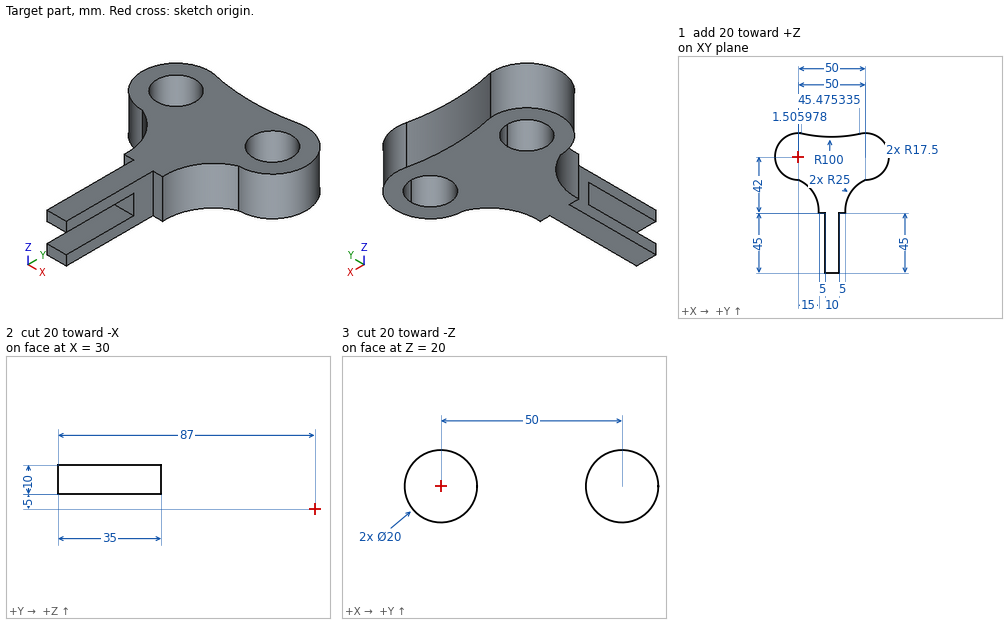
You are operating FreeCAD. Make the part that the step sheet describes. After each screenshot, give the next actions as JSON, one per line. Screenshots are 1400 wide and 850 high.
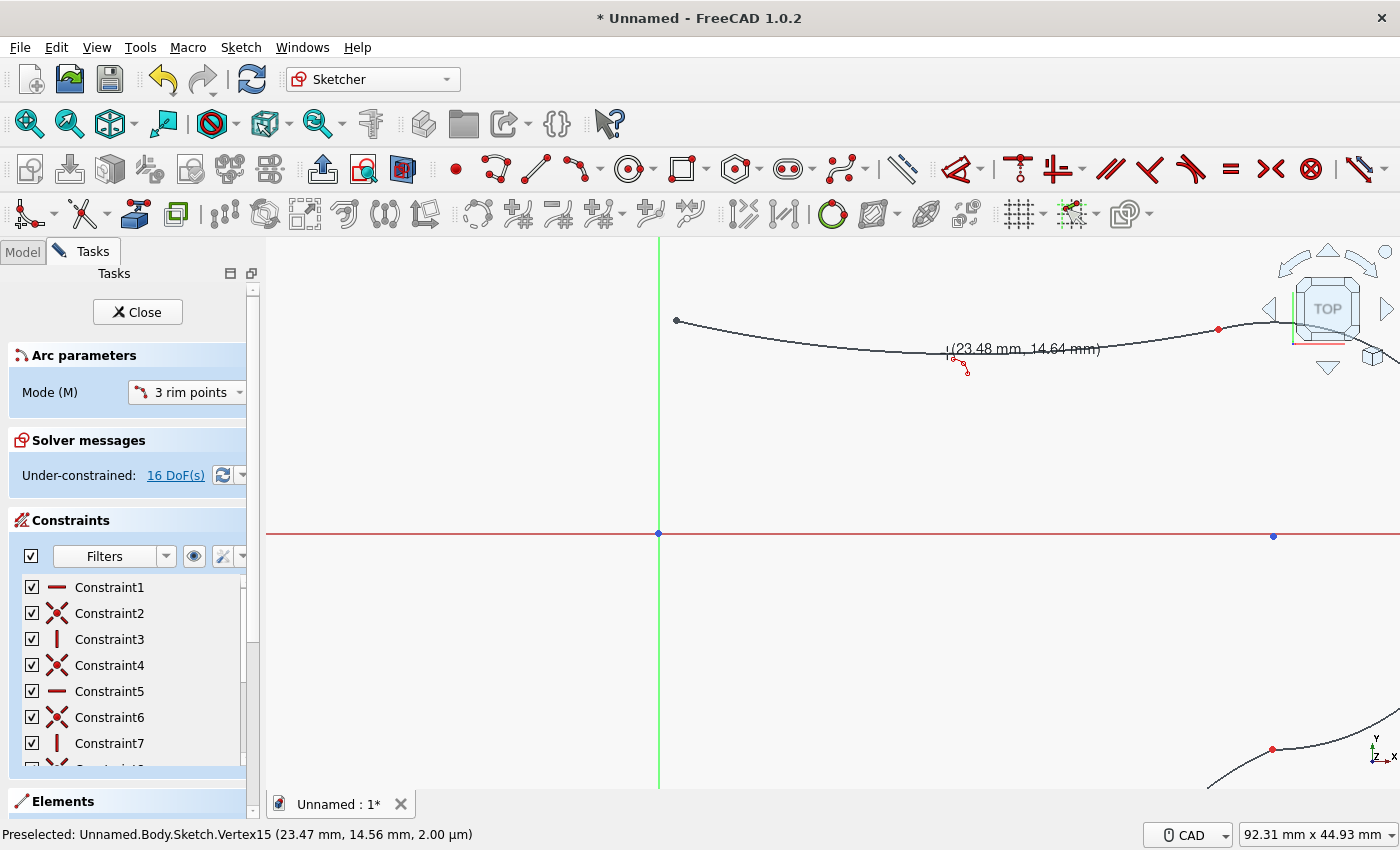
{"action": "left_click", "coordinate": [677, 321]}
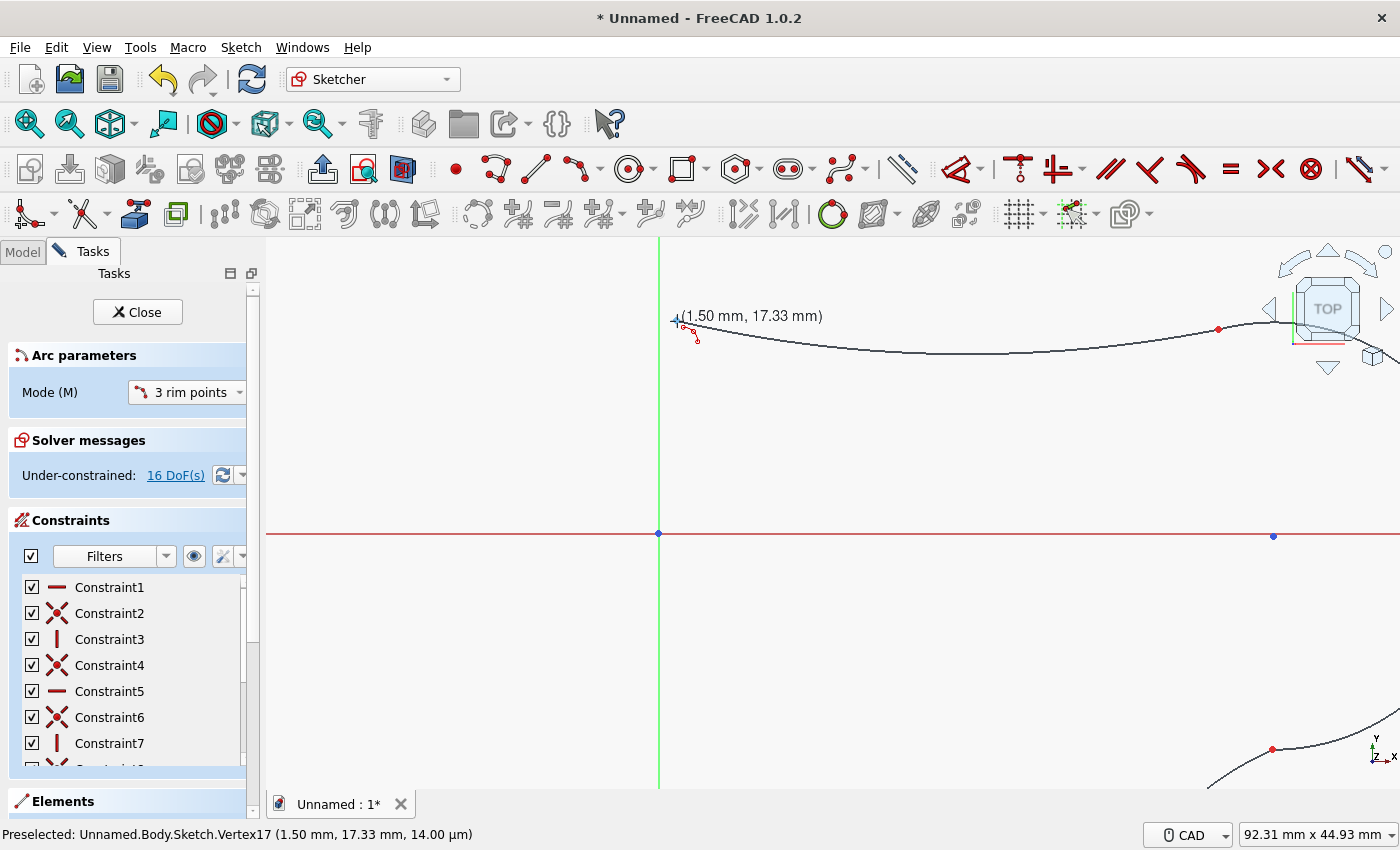
{"action": "scroll", "coordinate": [678, 320], "scroll_direction": "down", "scroll_amount": 6}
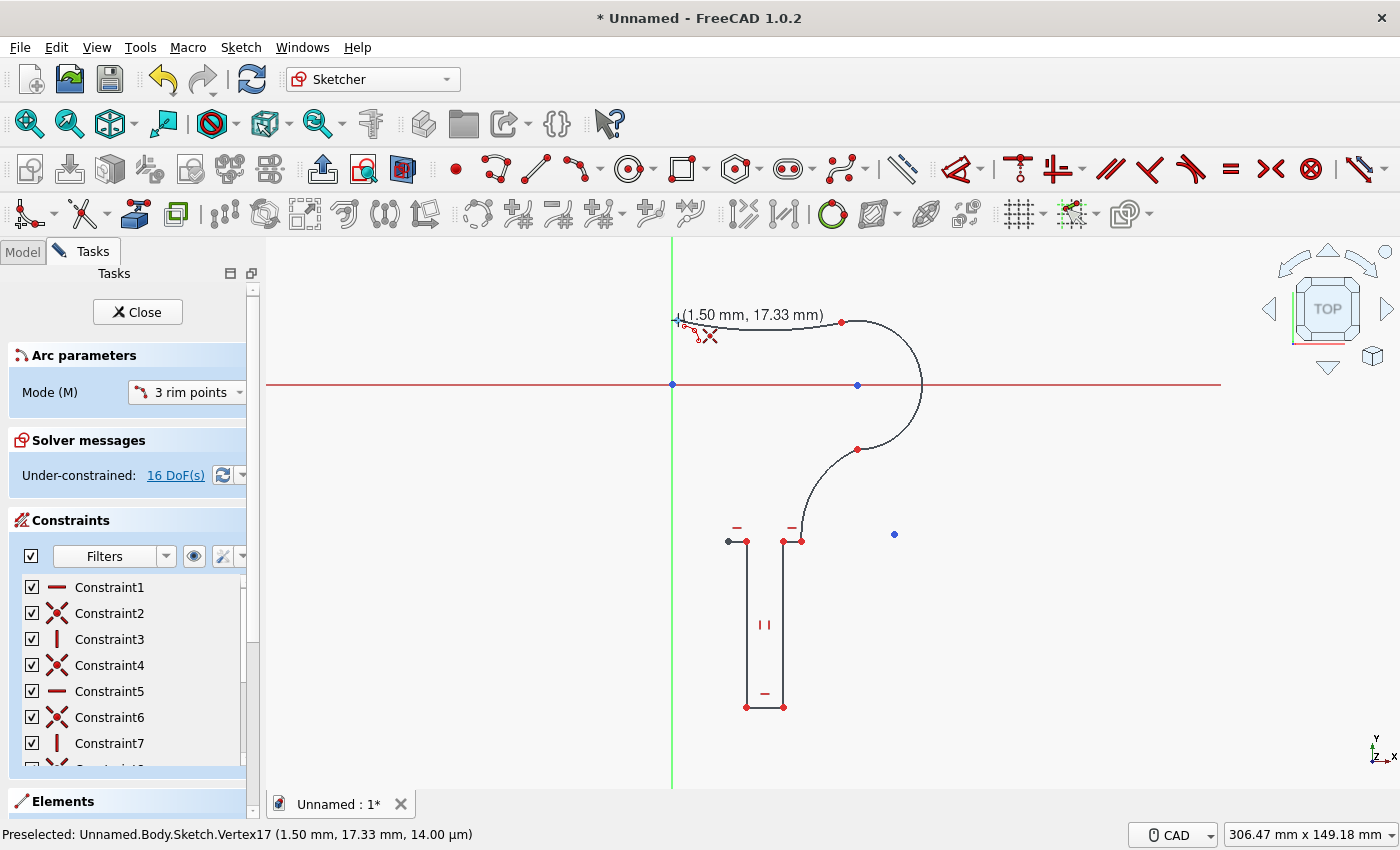
{"action": "left_click", "coordinate": [672, 449]}
{"action": "left_click", "coordinate": [612, 361]}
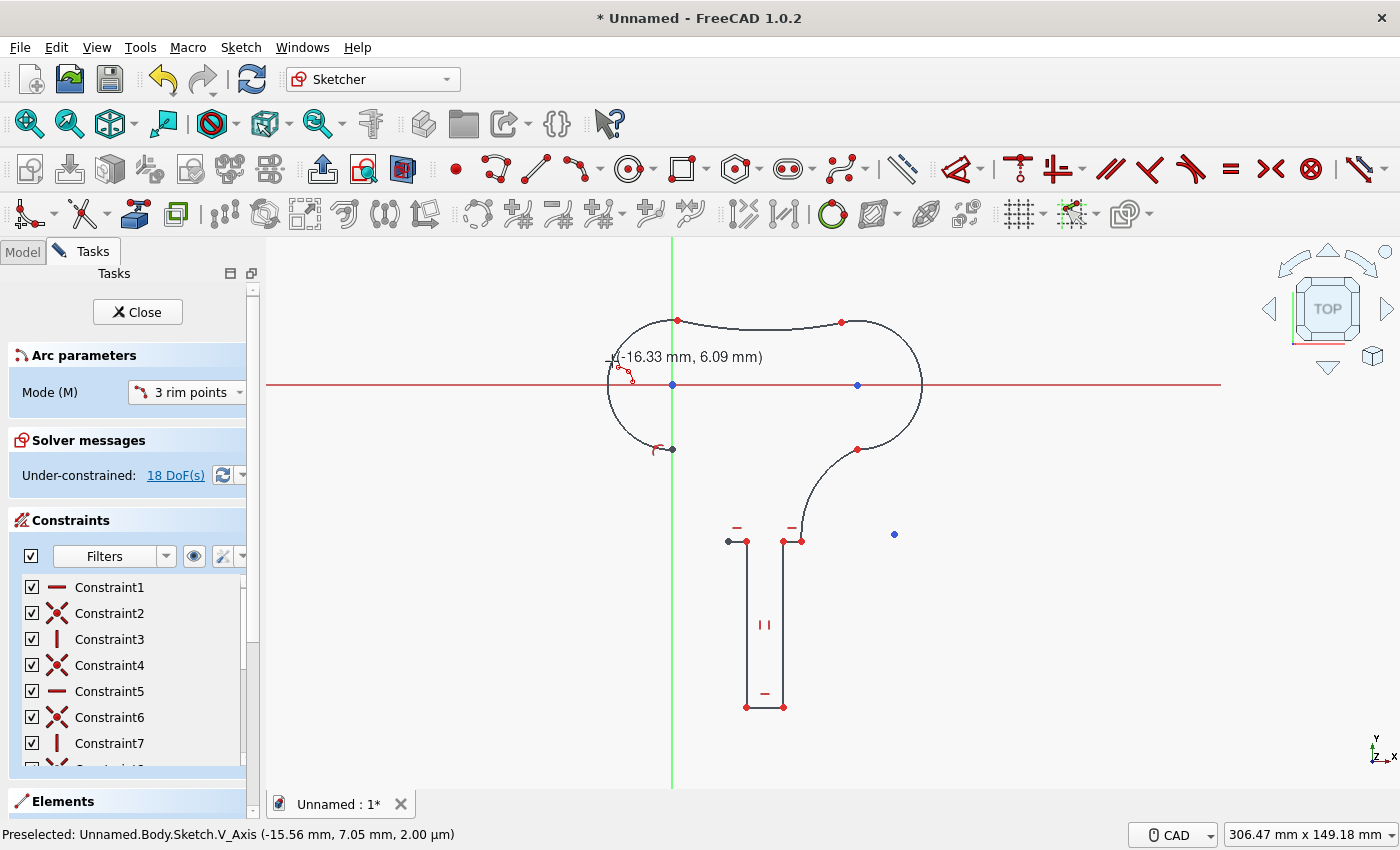
{"action": "left_click", "coordinate": [672, 450]}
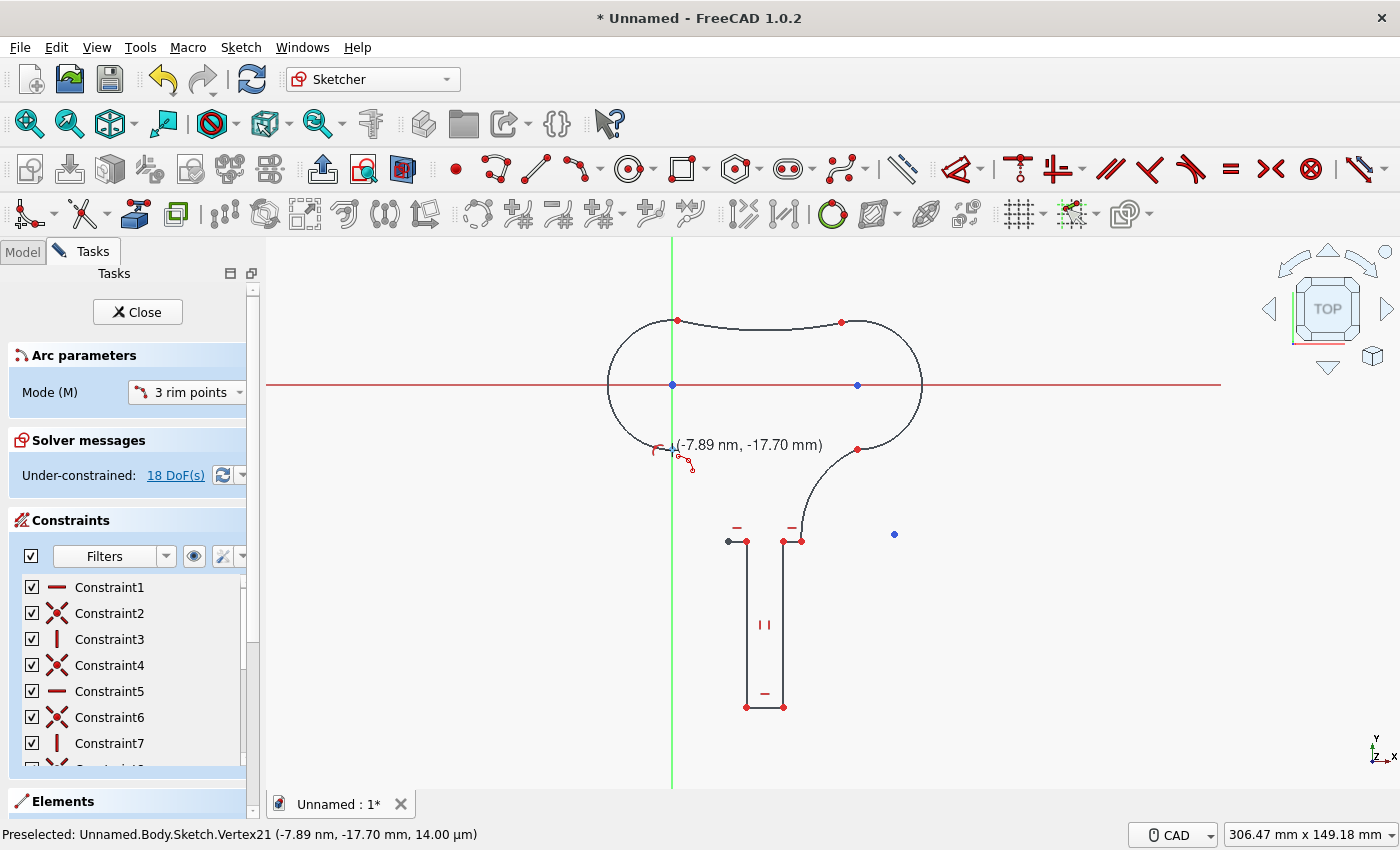
{"action": "scroll", "coordinate": [728, 540], "scroll_direction": "up", "scroll_amount": 3}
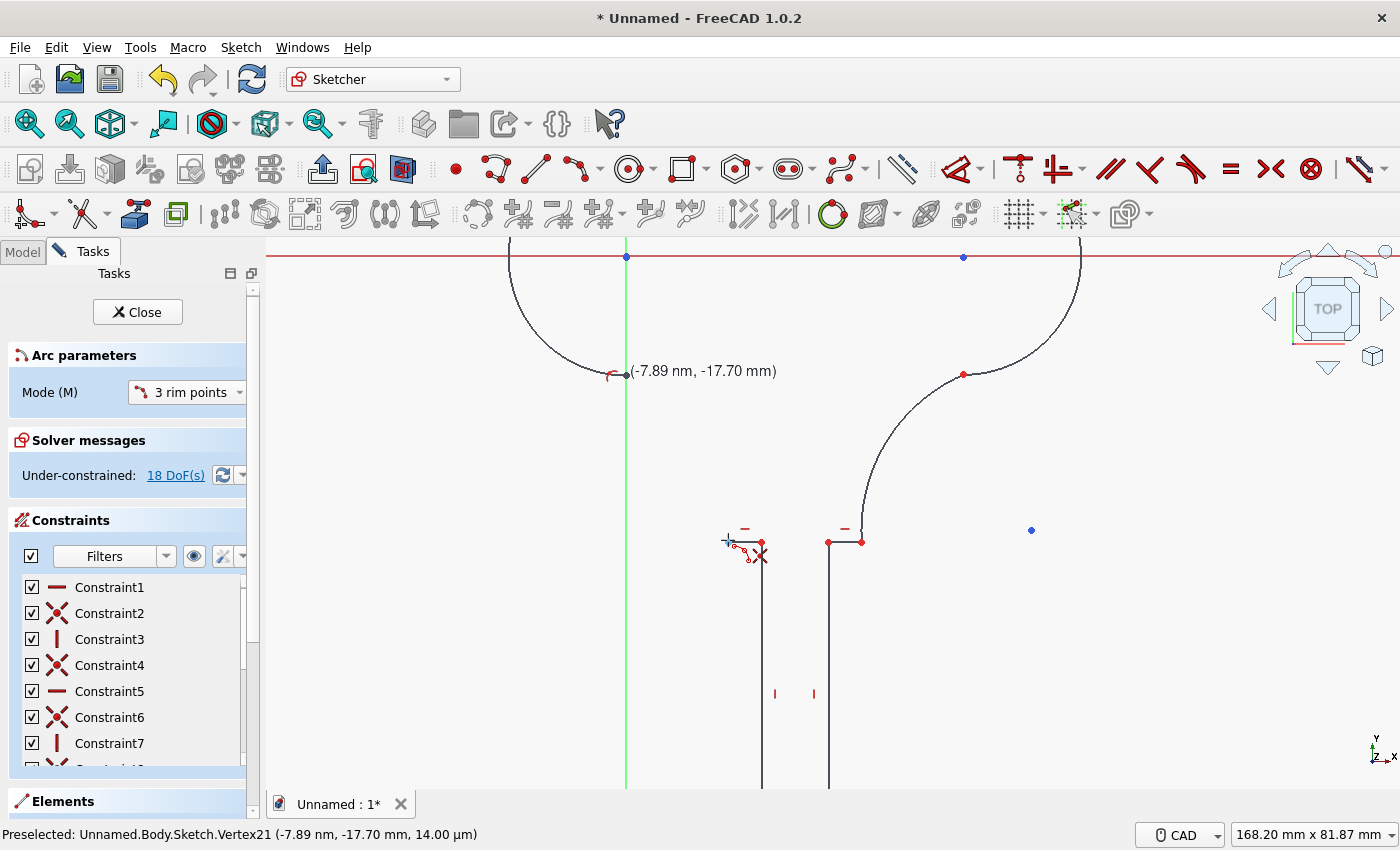
{"action": "left_click", "coordinate": [728, 542]}
{"action": "left_click", "coordinate": [703, 441]}
{"action": "key", "text": "Escape"}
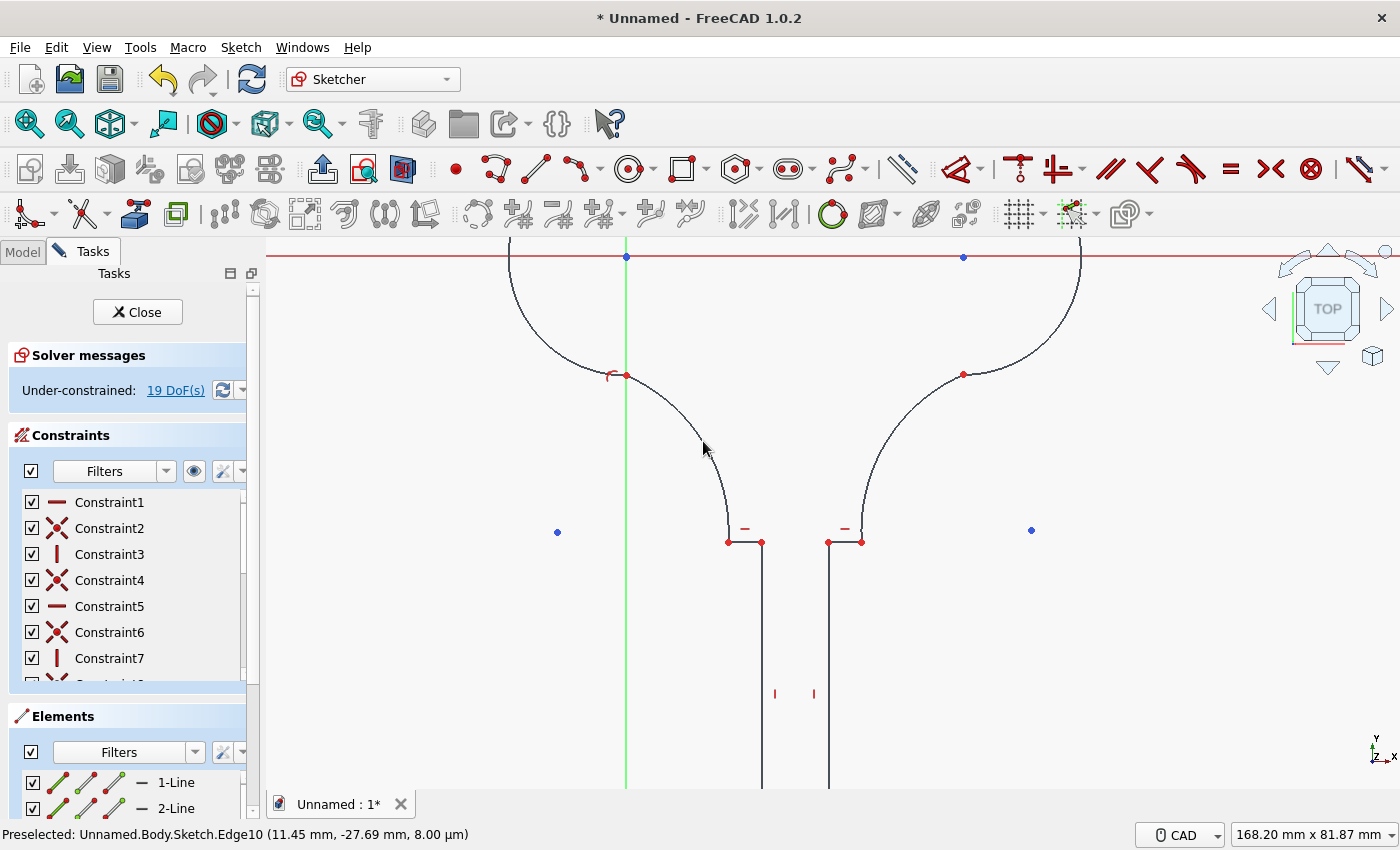
{"action": "scroll", "coordinate": [728, 540], "scroll_direction": "down", "scroll_amount": 3}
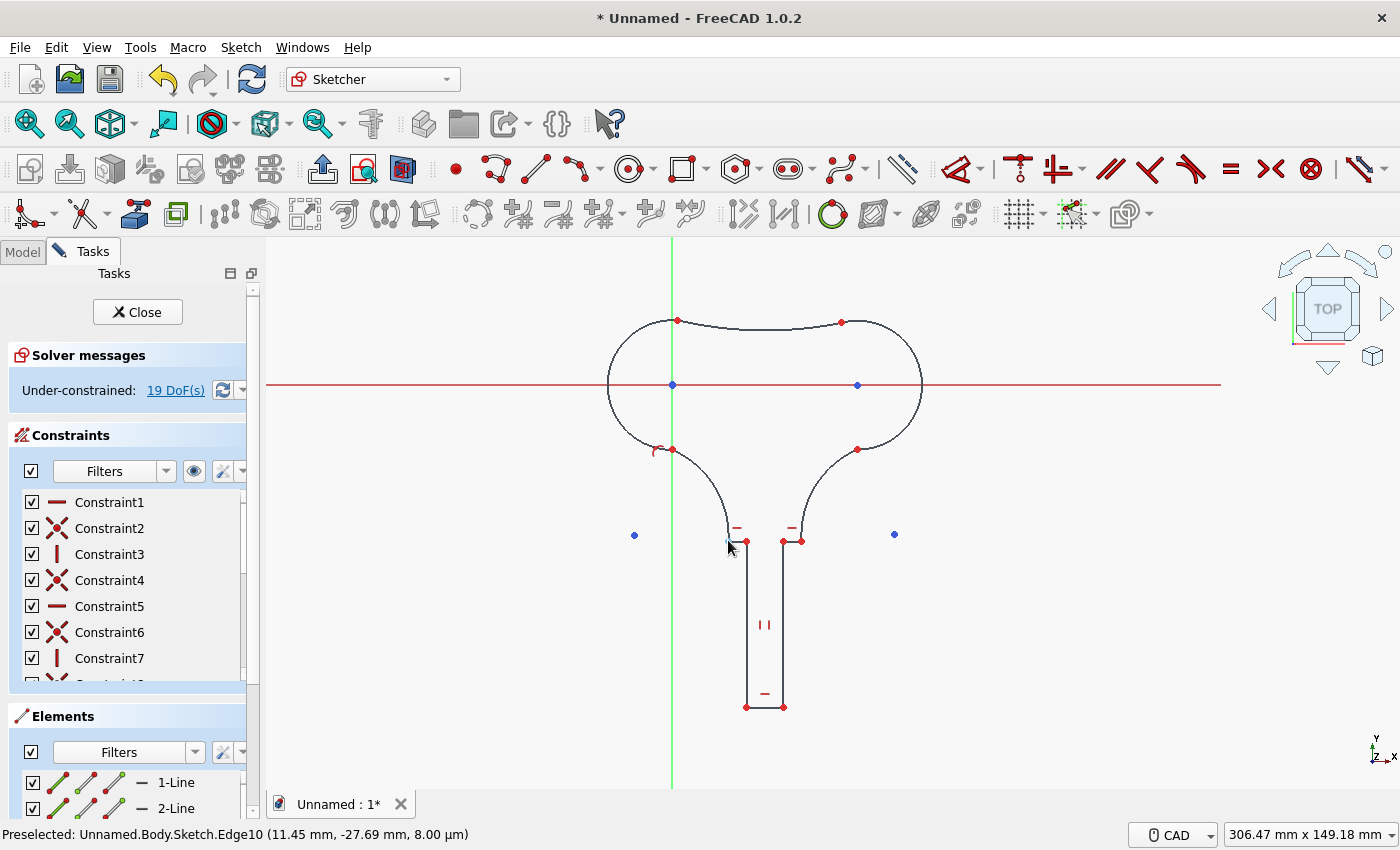
{"action": "left_click_drag", "start_coordinate": [662, 375], "coordinate": [683, 395]}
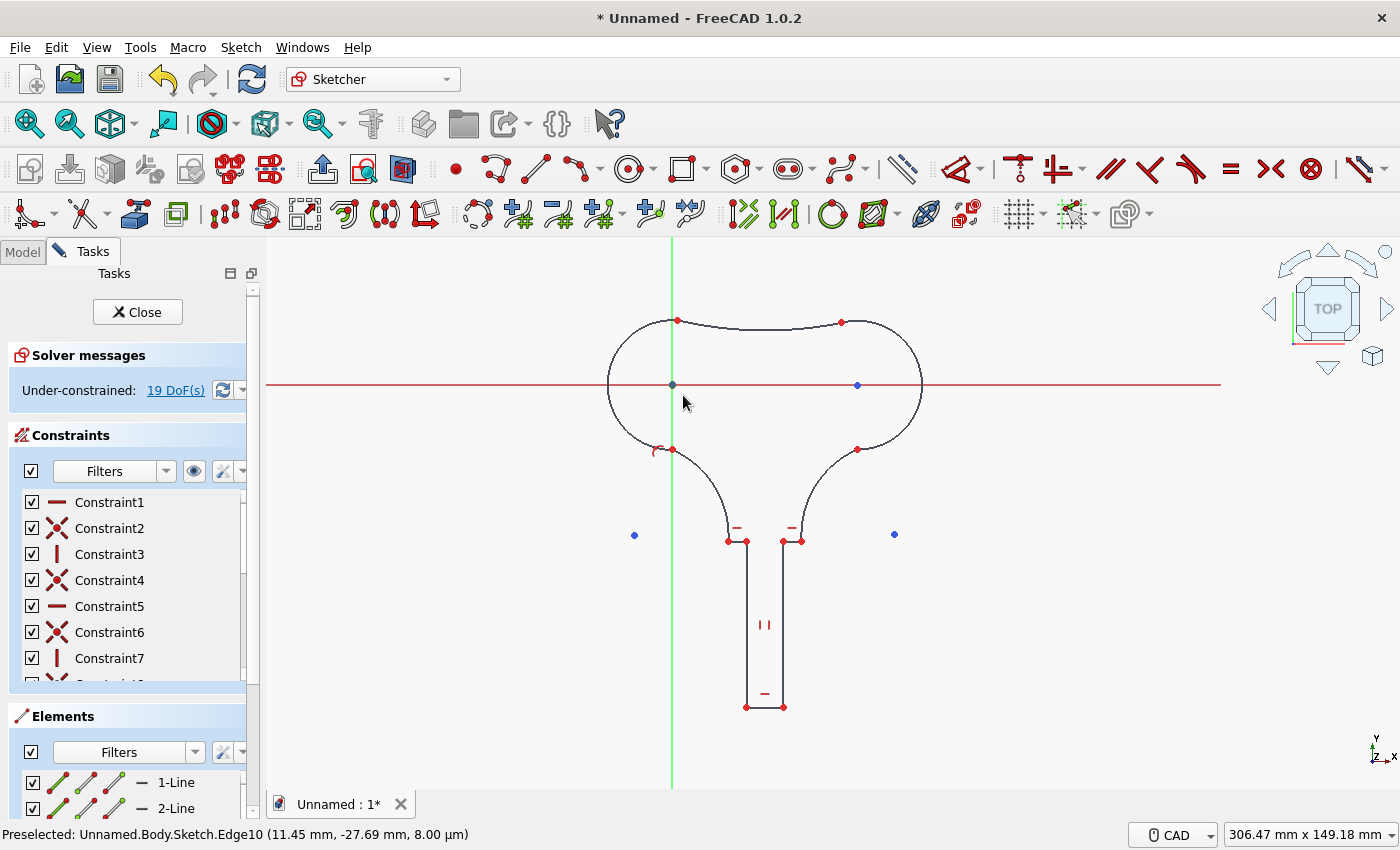
{"action": "left_click", "coordinate": [1018, 170]}